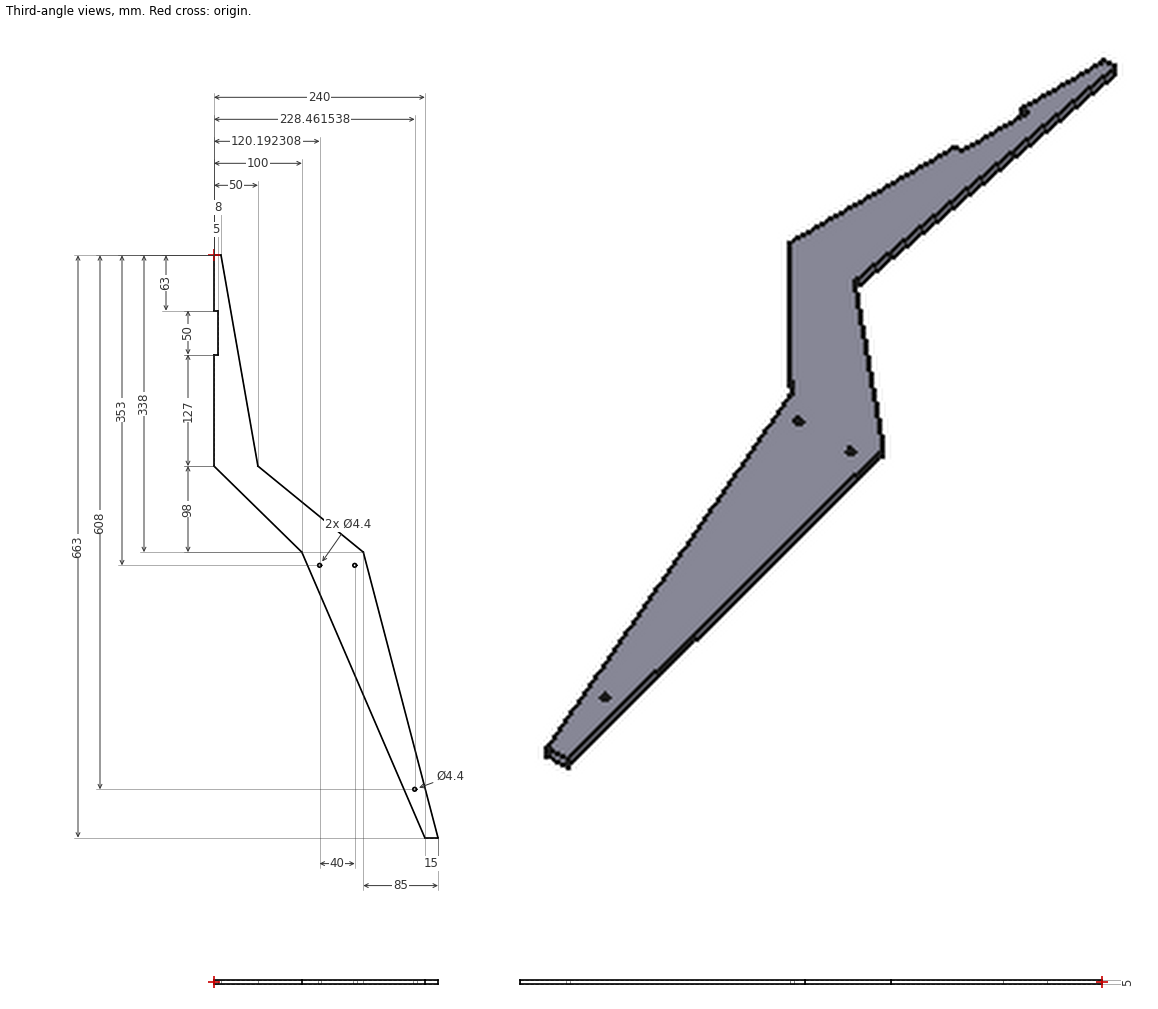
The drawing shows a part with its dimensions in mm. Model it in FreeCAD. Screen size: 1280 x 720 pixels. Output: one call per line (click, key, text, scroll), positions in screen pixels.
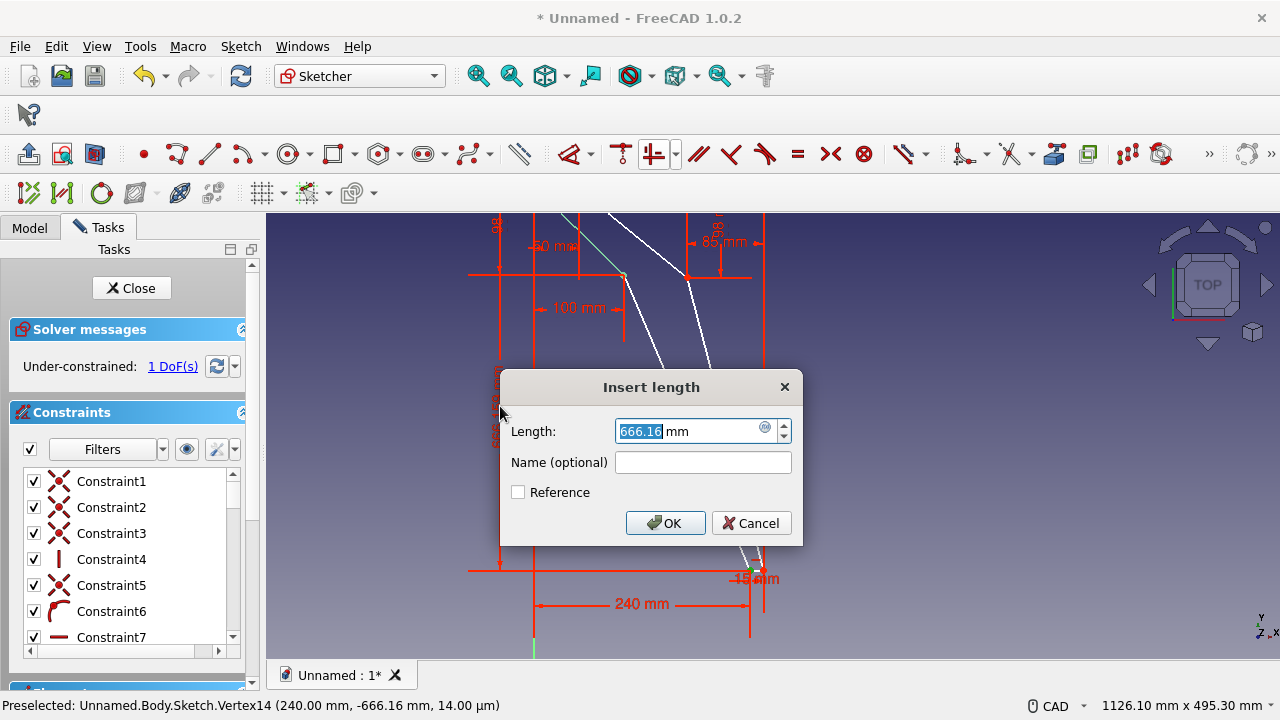
text(663)
key(Return)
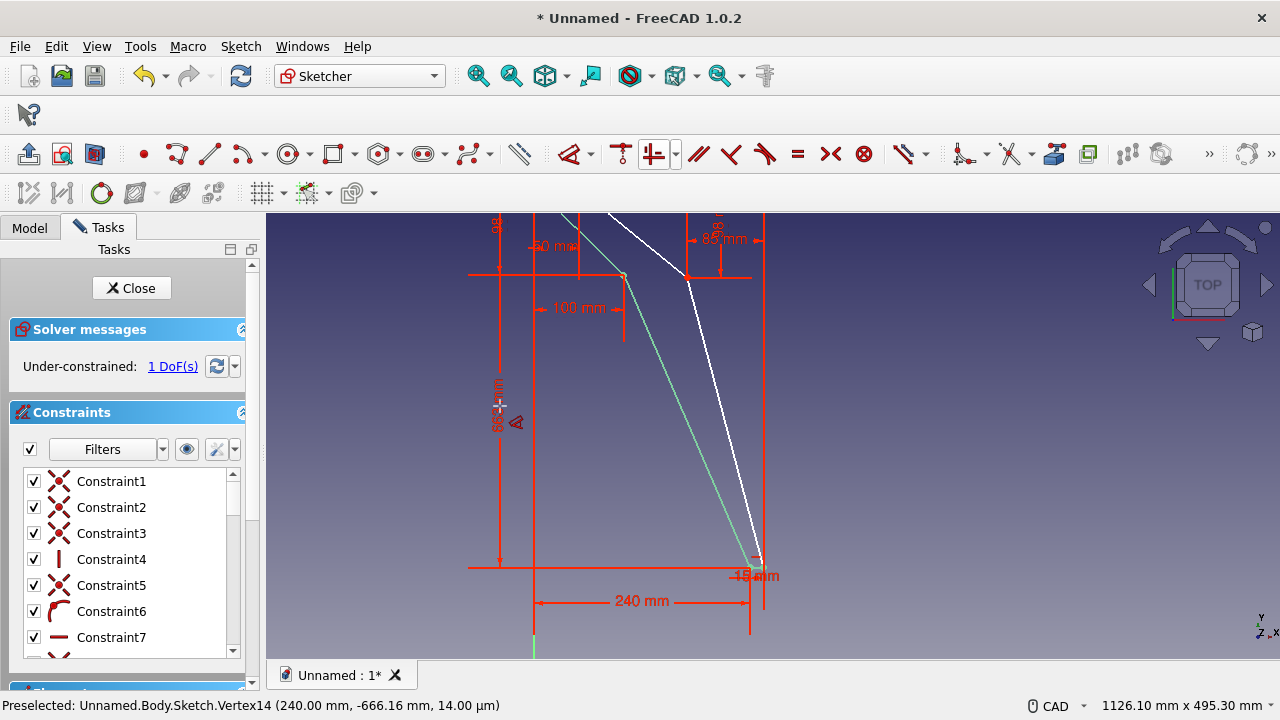
click(687, 278)
click(500, 272)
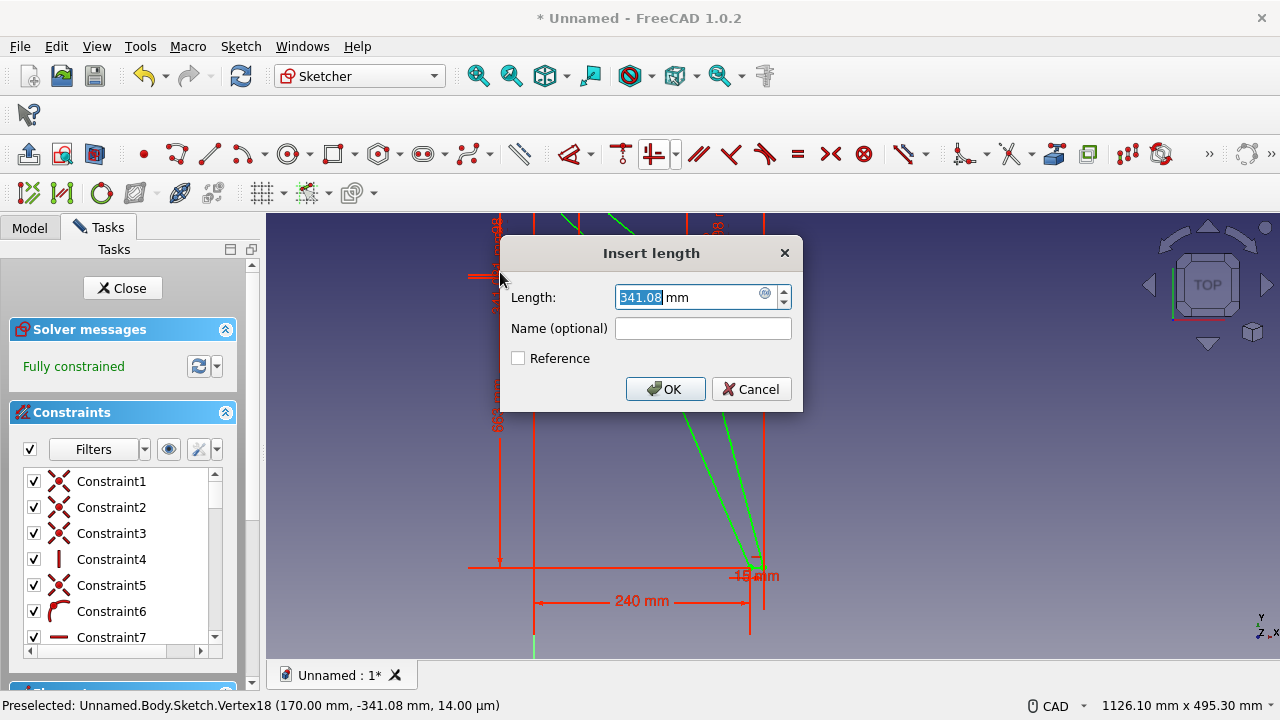
text(338)
key(Return)
key(Escape)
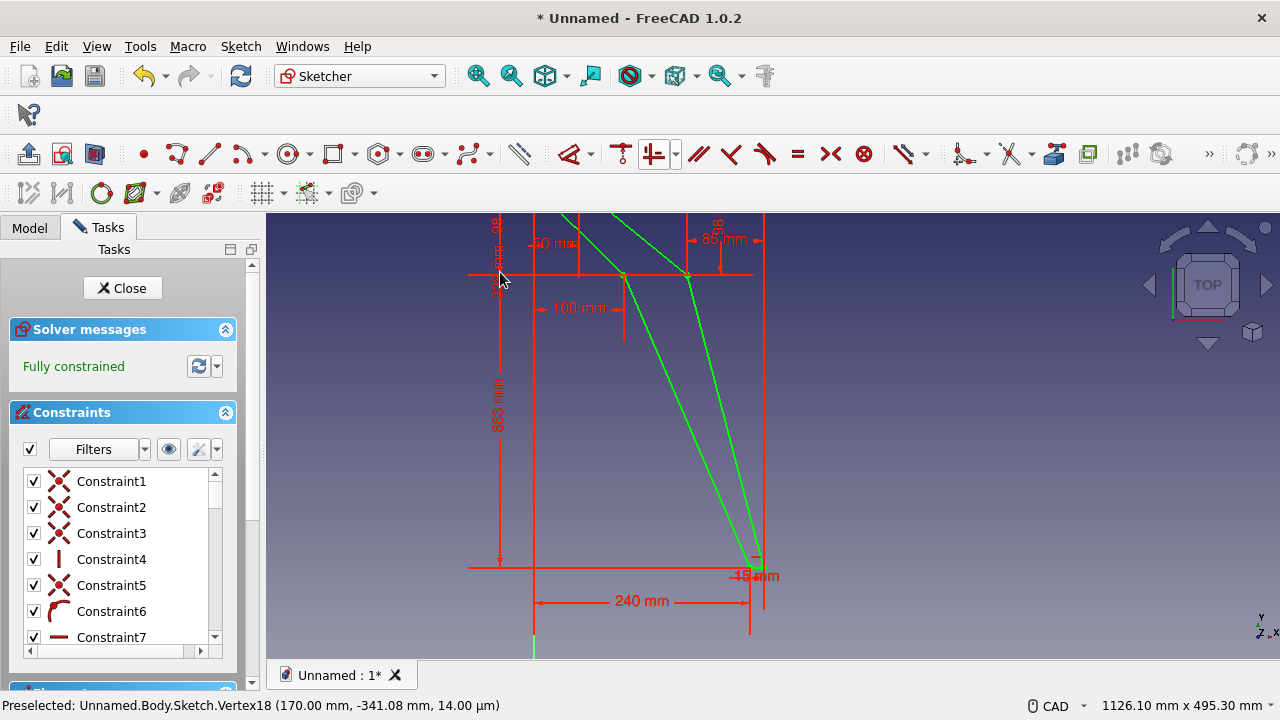
click(123, 288)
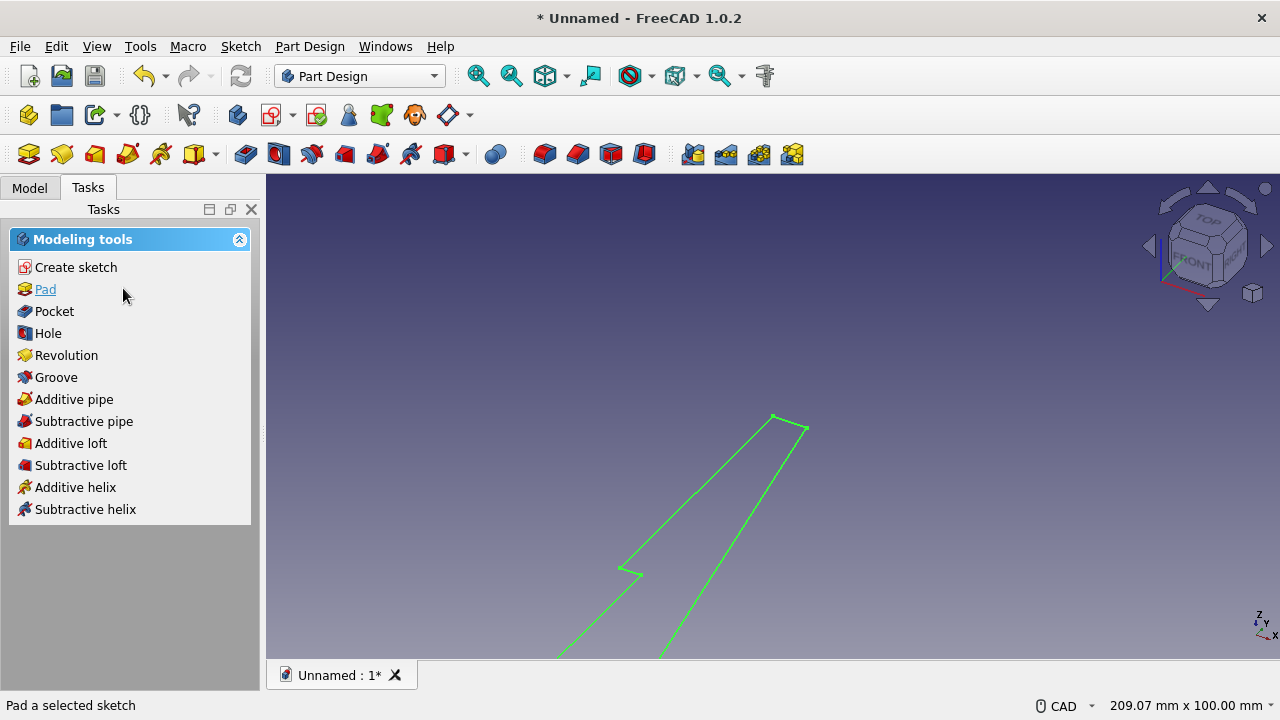
click(29, 154)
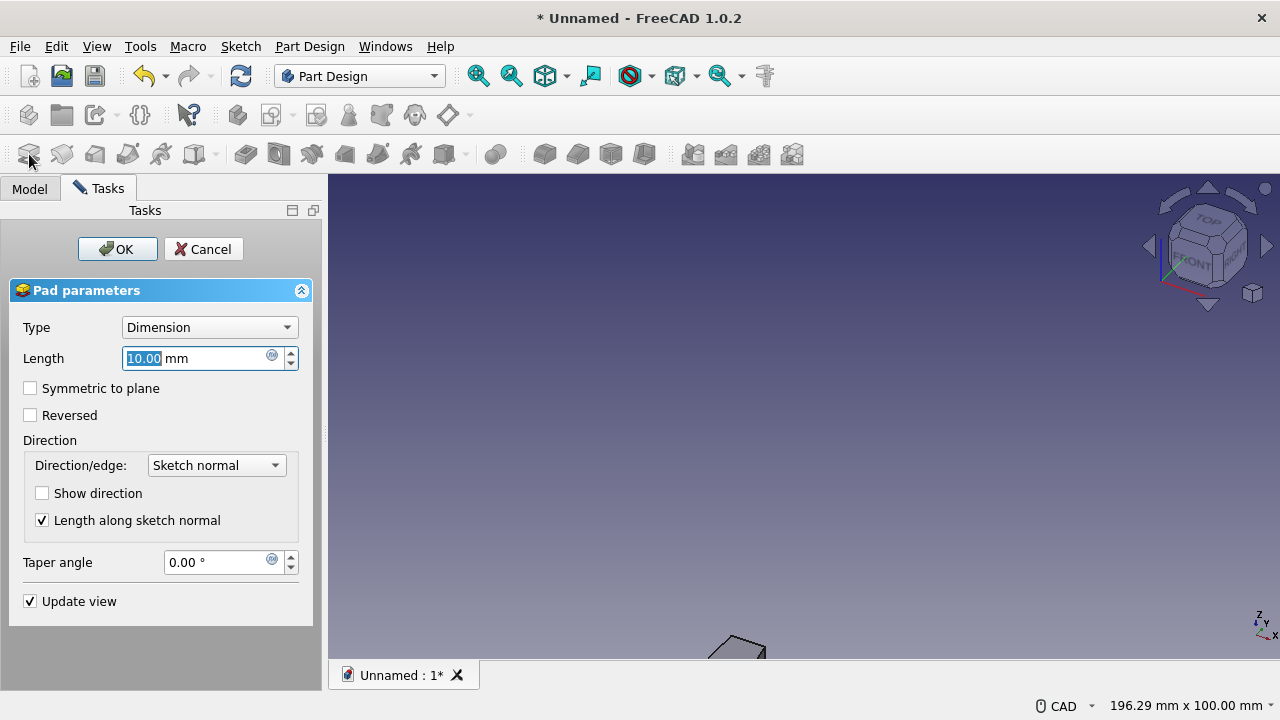
text(5)
key(Tab)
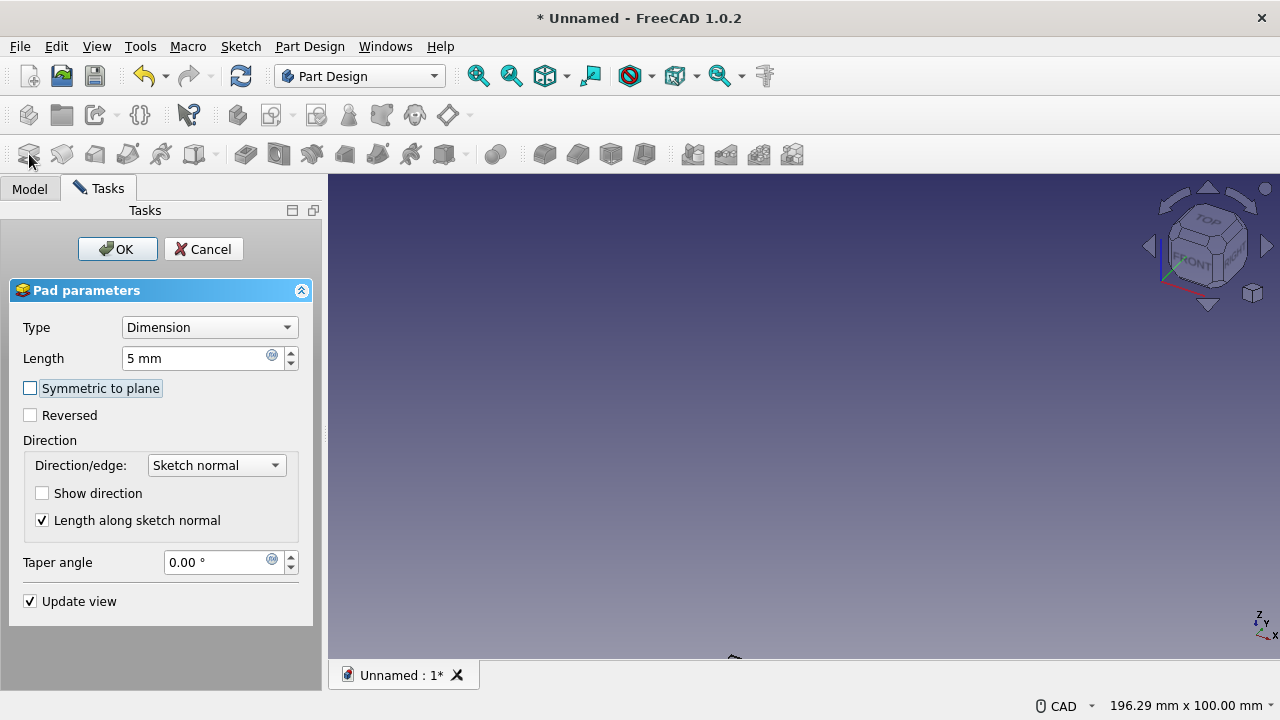
click(31, 388)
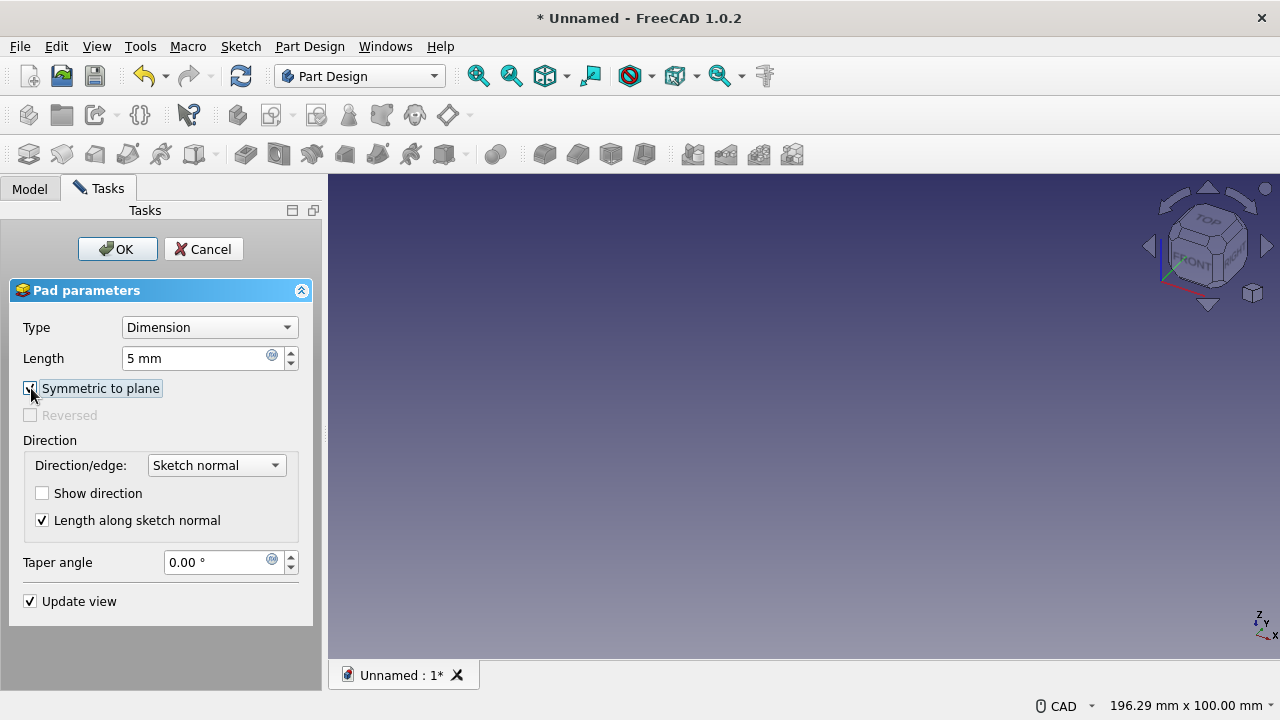
click(118, 249)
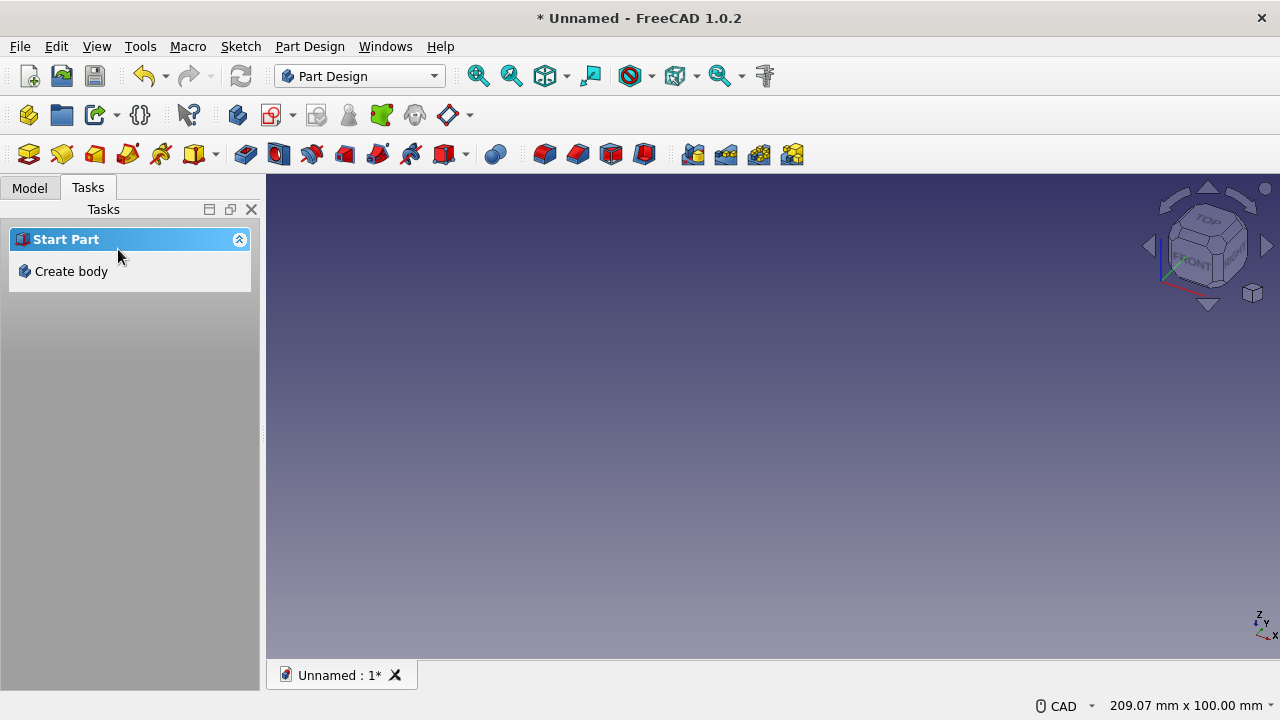
click(479, 76)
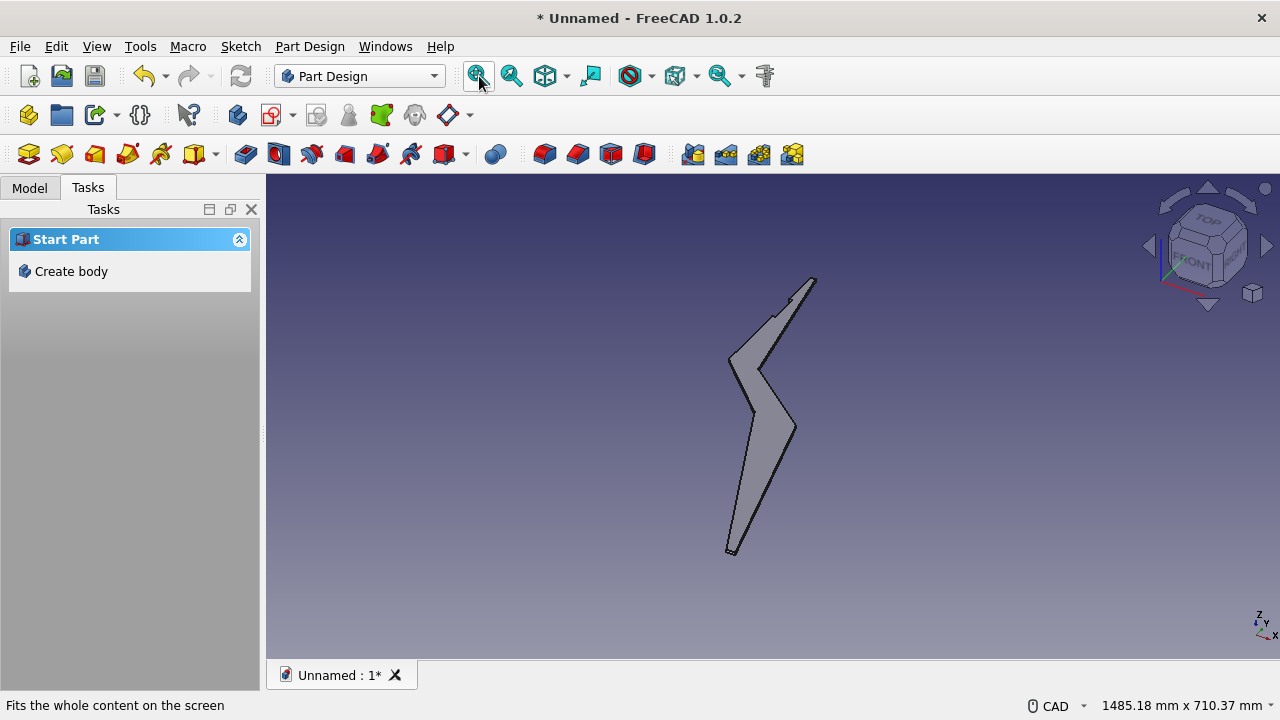
click(762, 453)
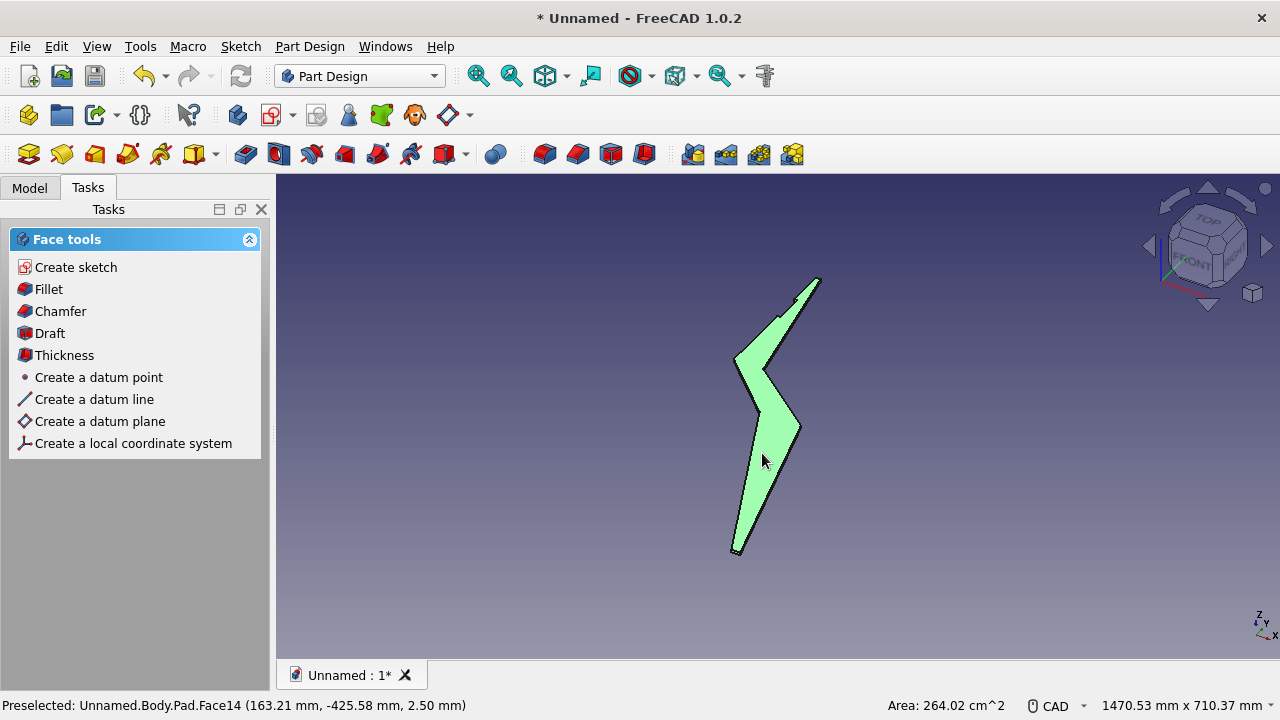
click(270, 116)